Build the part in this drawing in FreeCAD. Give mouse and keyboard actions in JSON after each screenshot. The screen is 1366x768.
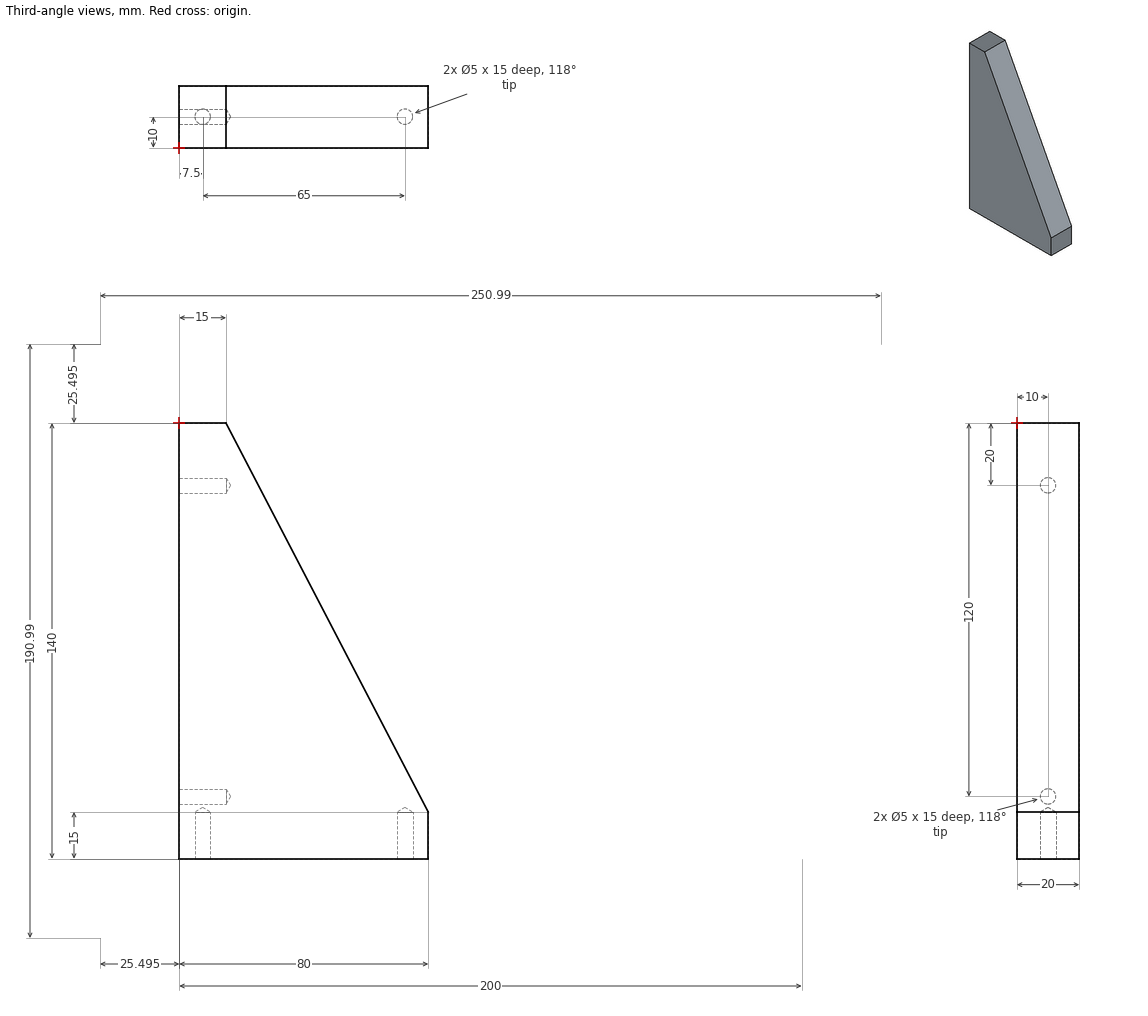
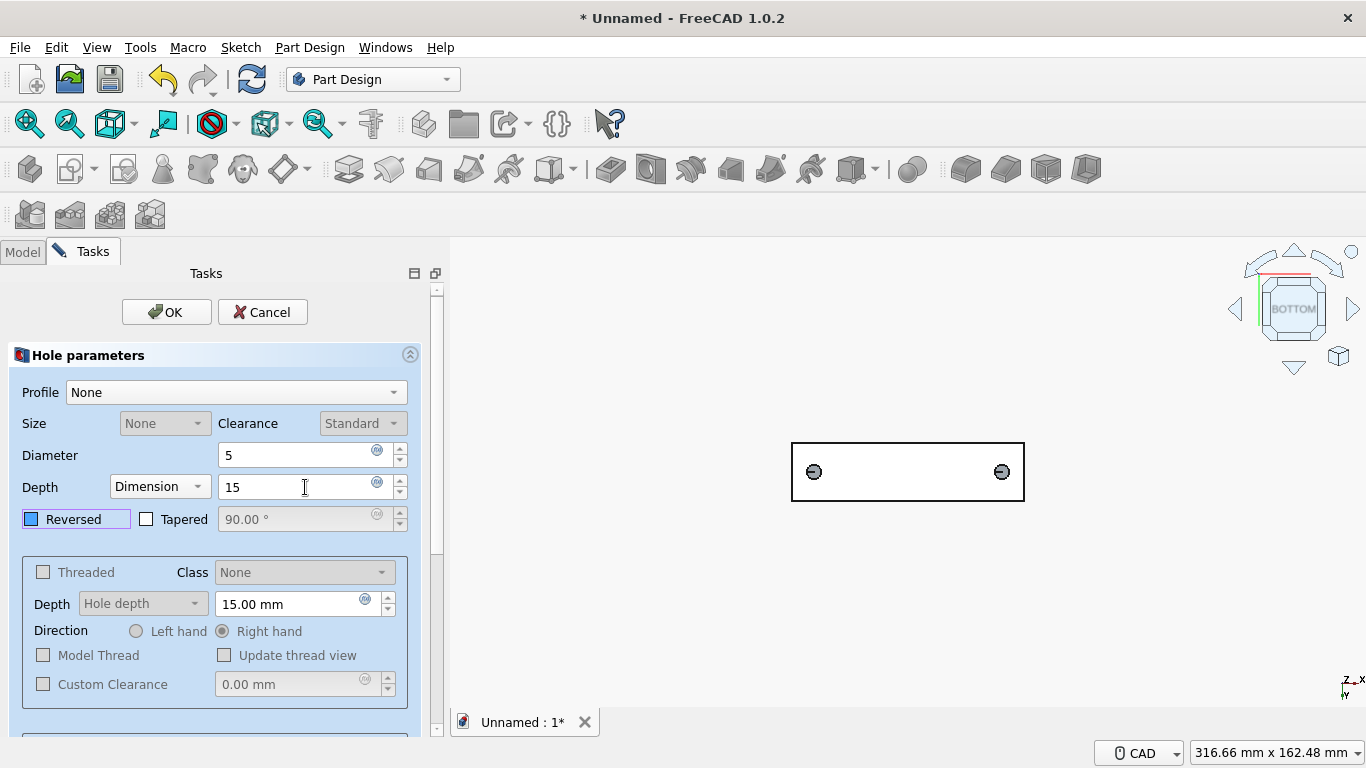
{"action": "left_click", "coordinate": [167, 312]}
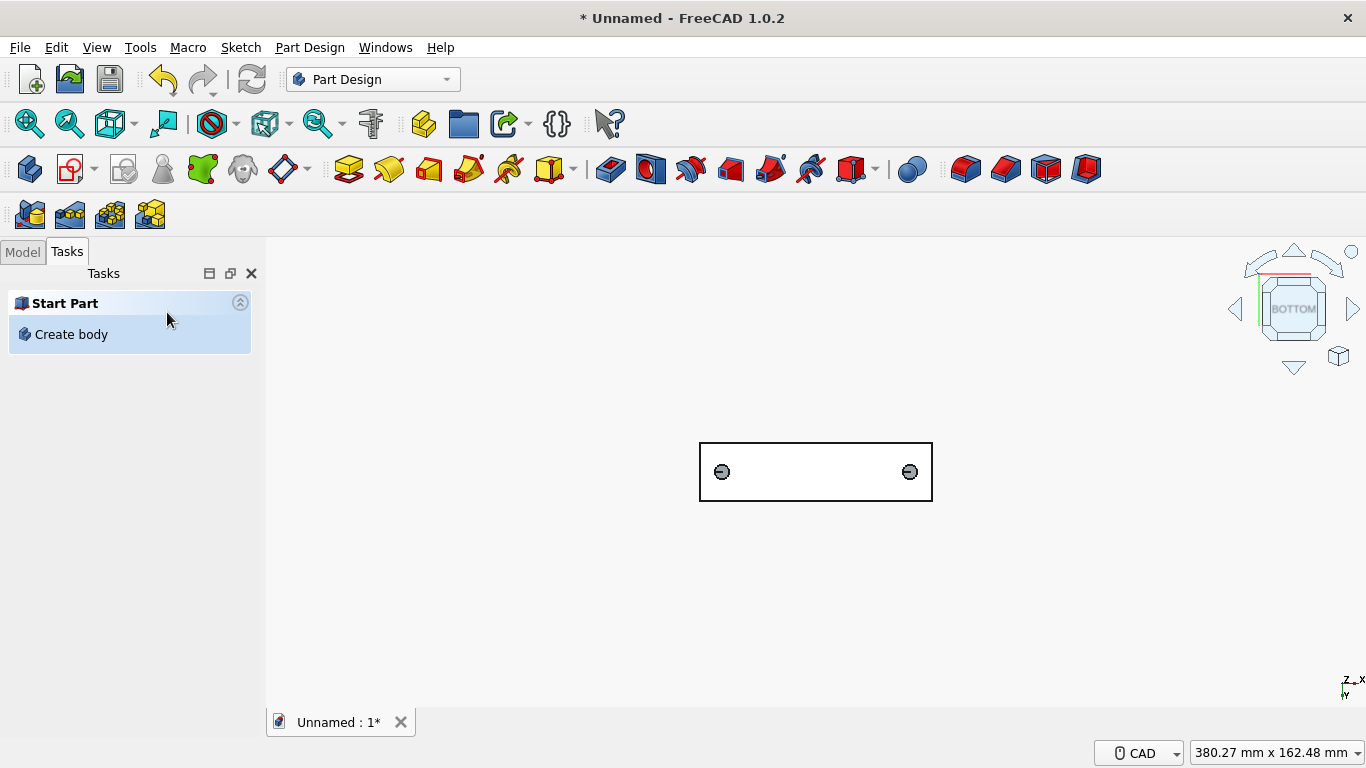
{"action": "key", "text": "0"}